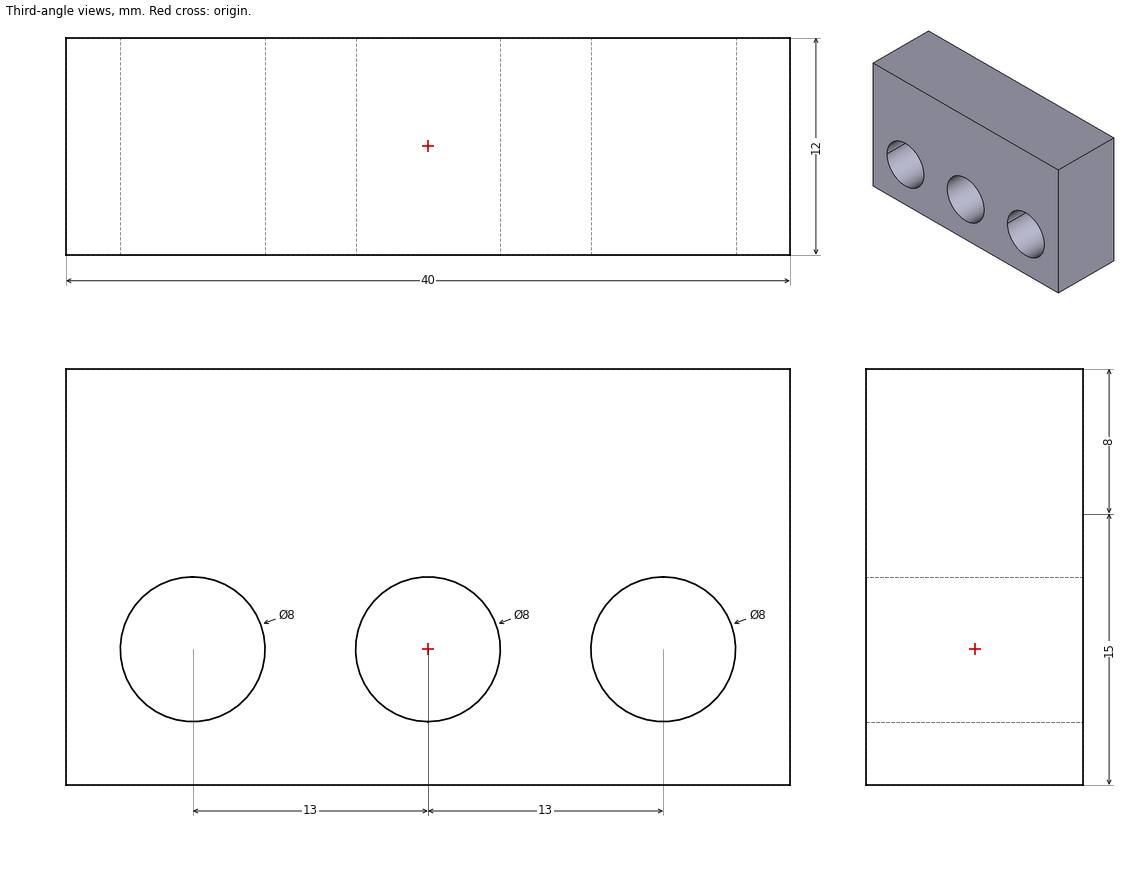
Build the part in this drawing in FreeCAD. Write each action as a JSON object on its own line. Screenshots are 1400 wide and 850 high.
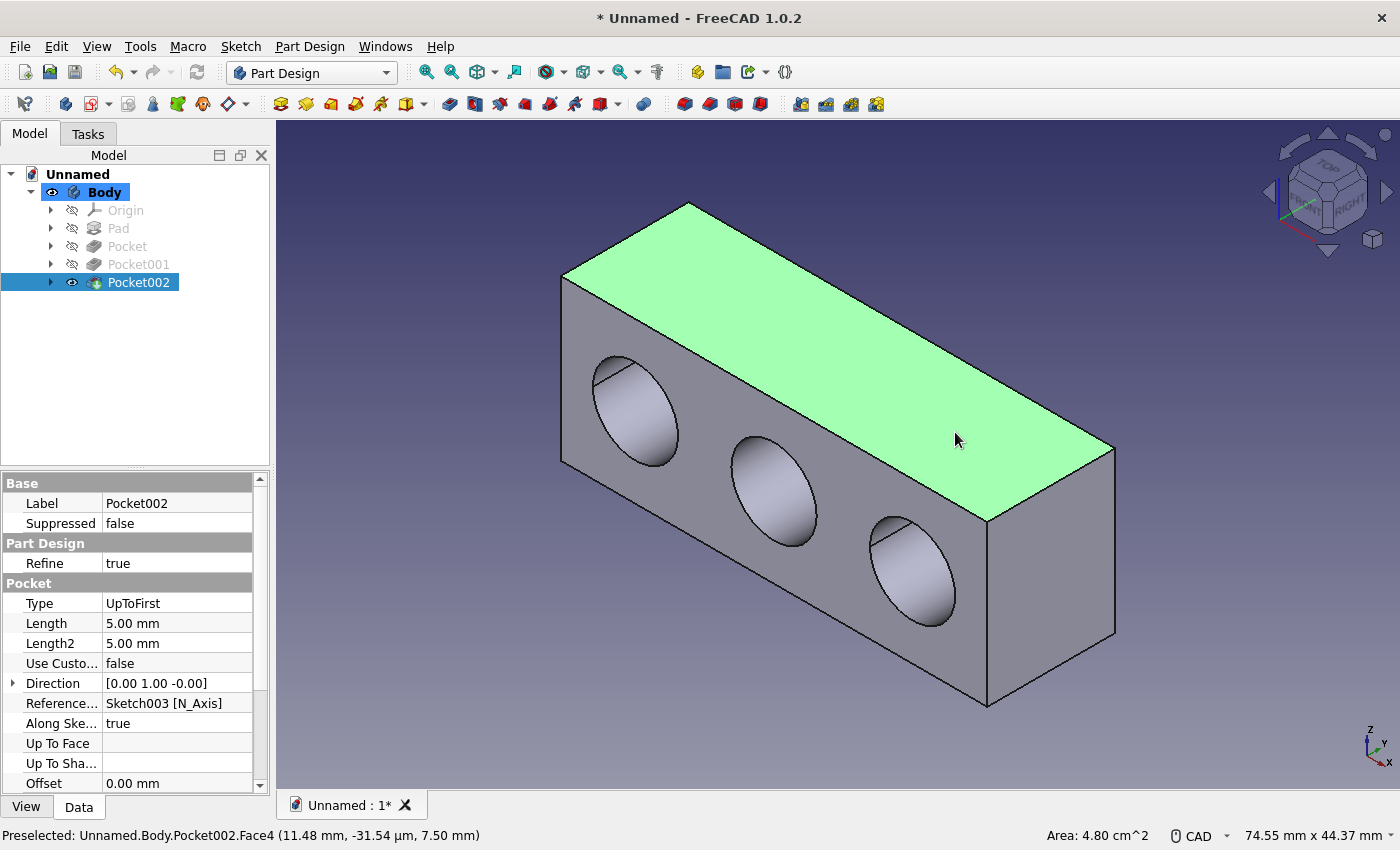
{"action": "left_click", "coordinate": [90, 104]}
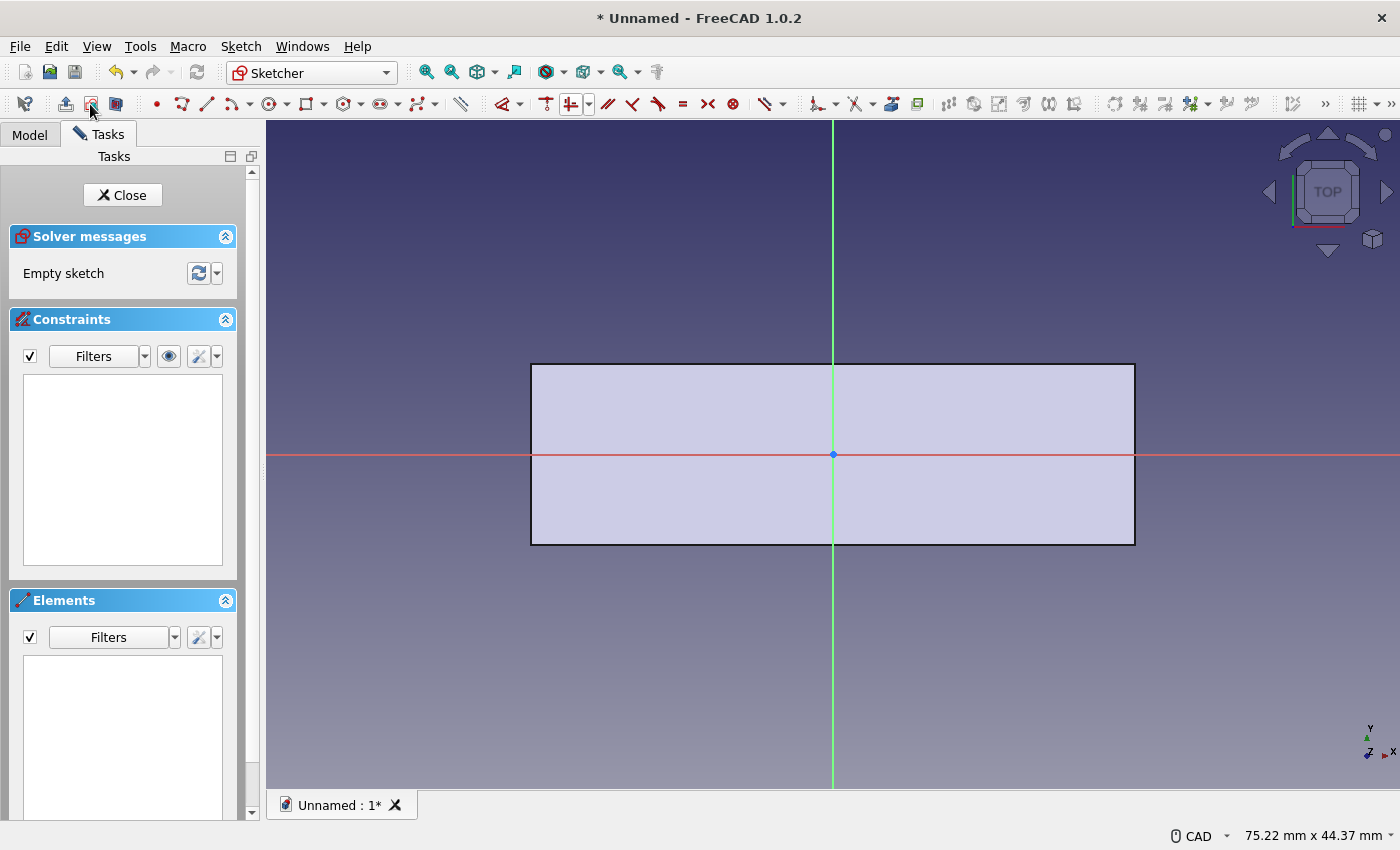
{"action": "key", "text": "g v"}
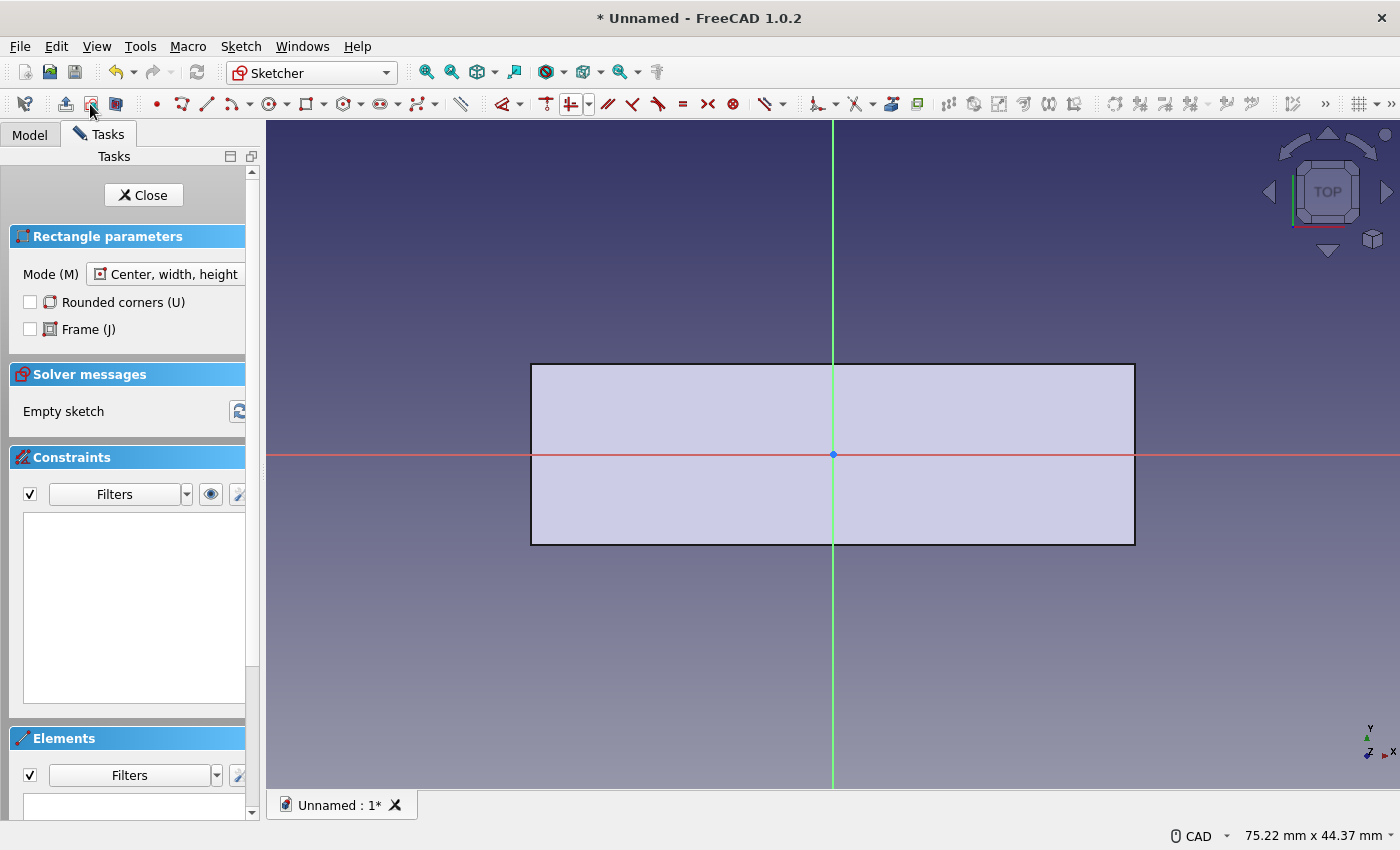
{"action": "left_click", "coordinate": [833, 454]}
{"action": "left_click", "coordinate": [1135, 364]}
{"action": "key", "text": "Escape"}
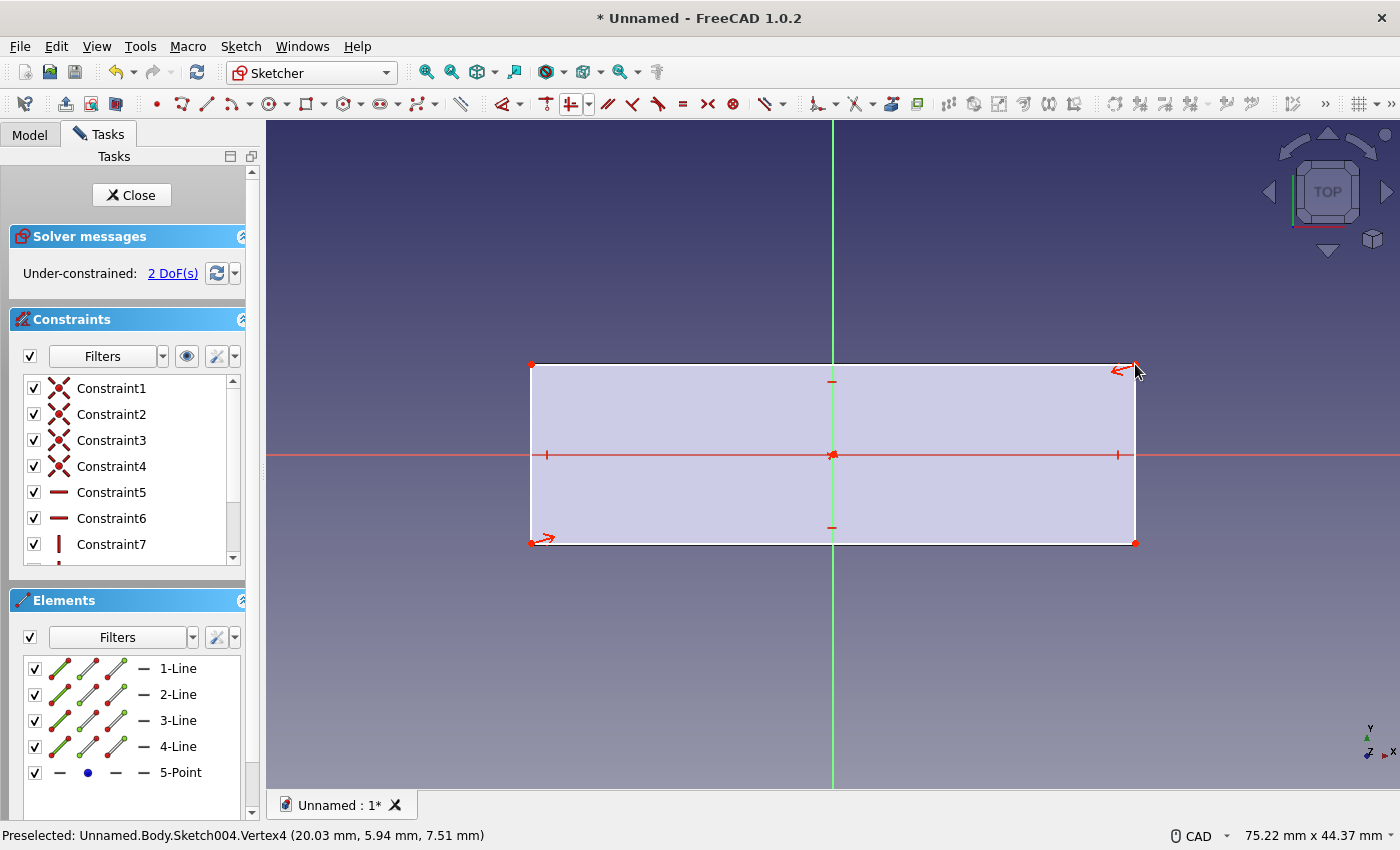
{"action": "left_click", "coordinate": [502, 104]}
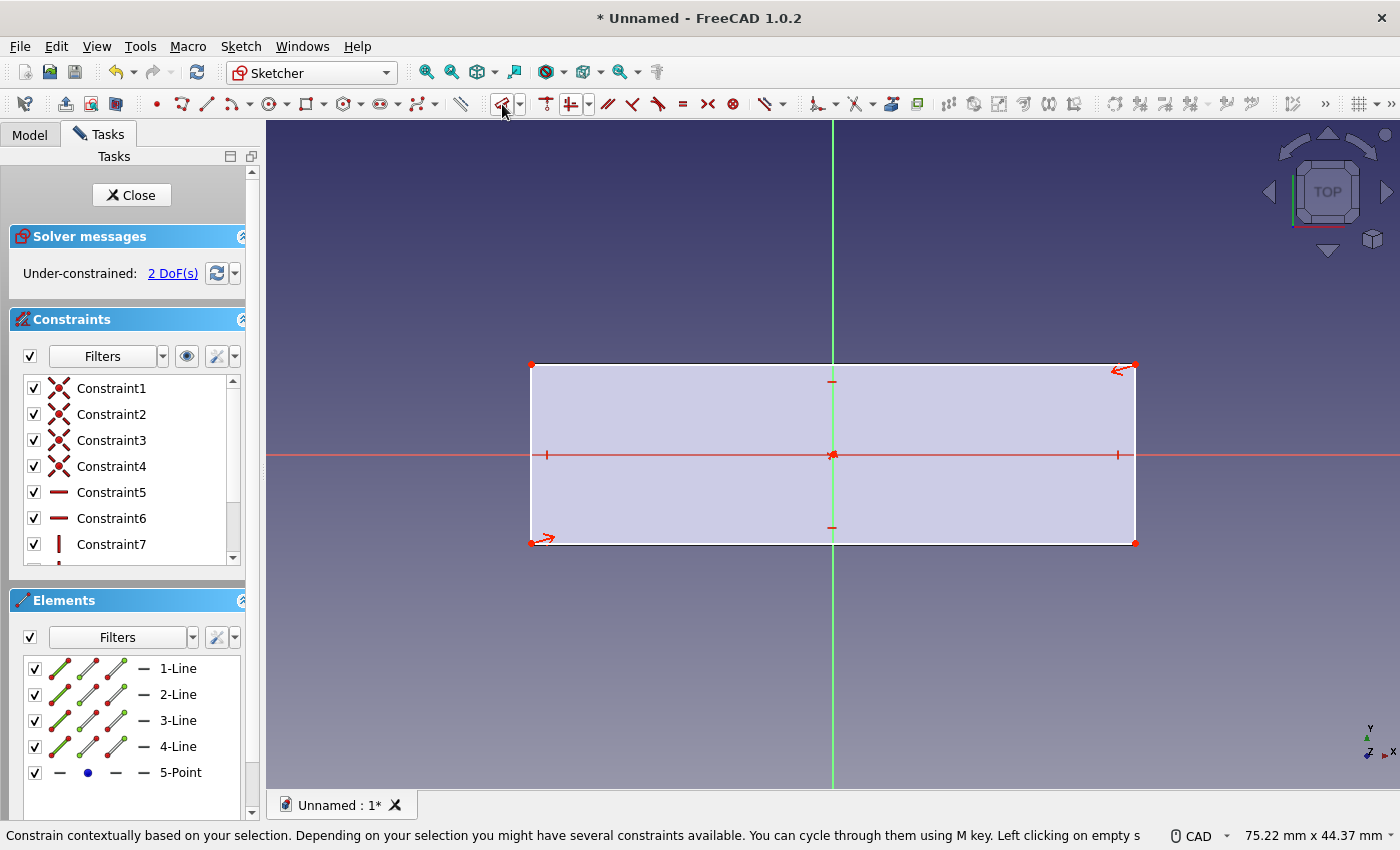
{"action": "left_click", "coordinate": [712, 544]}
{"action": "left_click", "coordinate": [694, 578]}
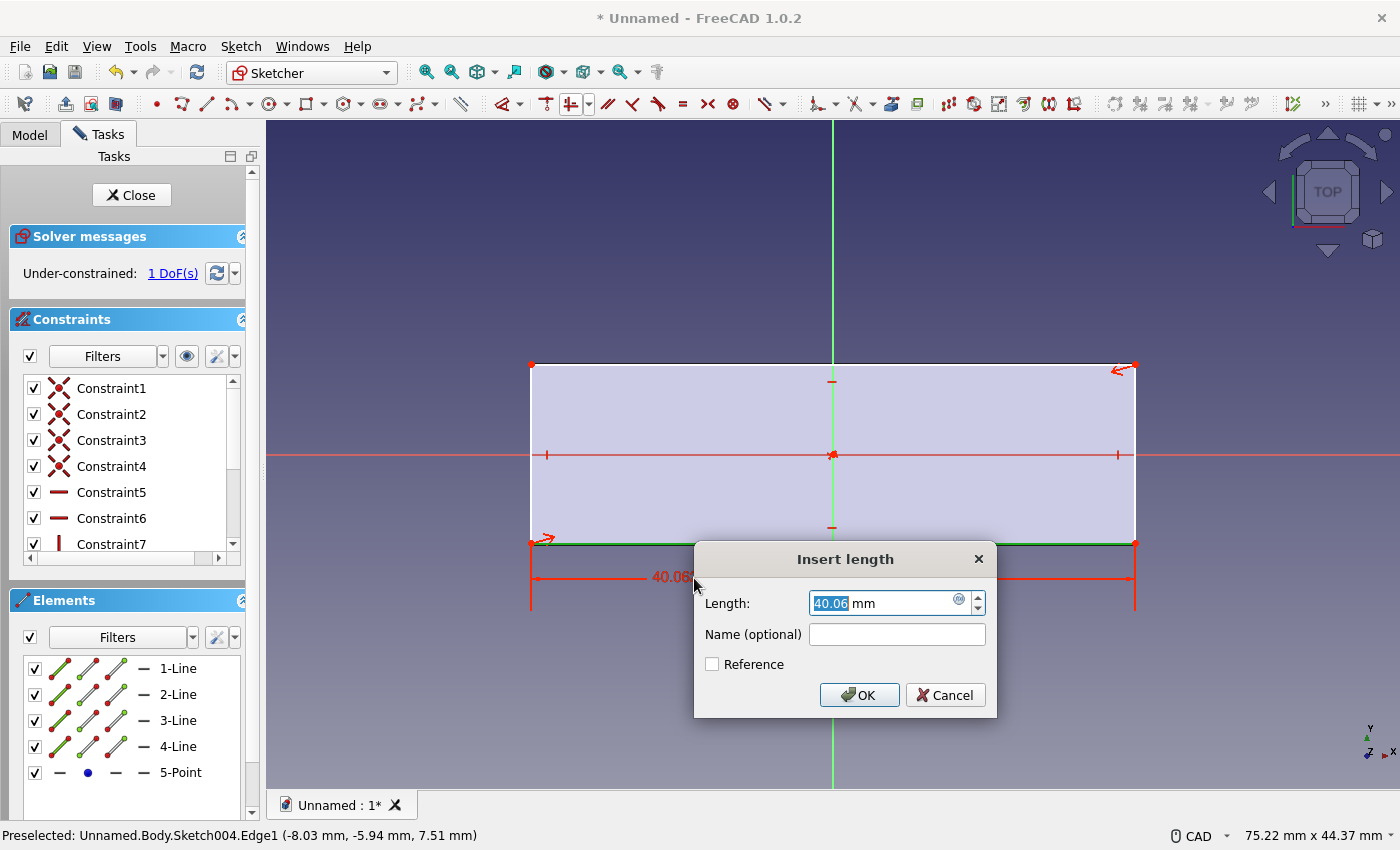
{"action": "type", "text": "40"}
{"action": "key", "text": "Return"}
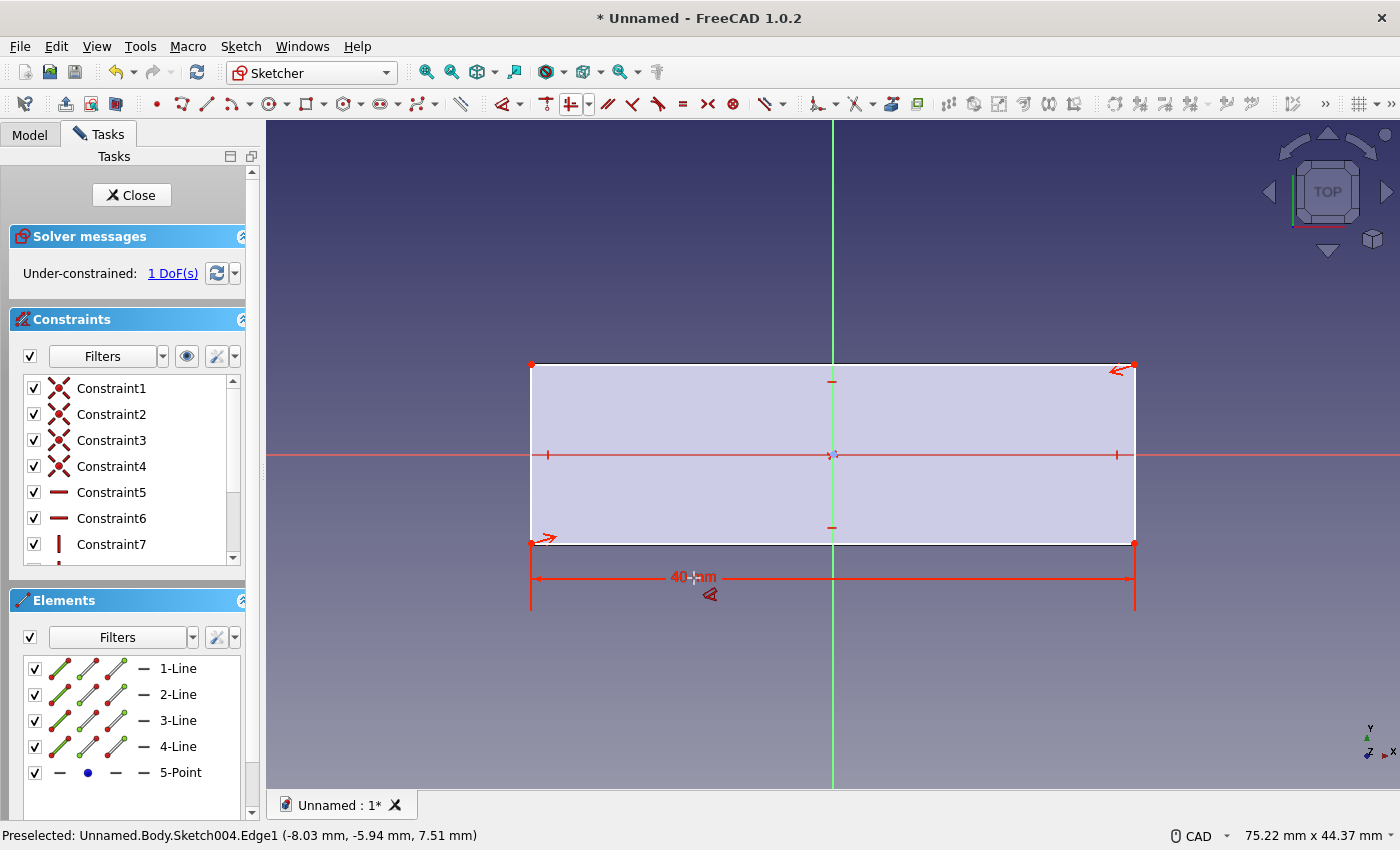
{"action": "left_click", "coordinate": [1135, 490]}
{"action": "left_click", "coordinate": [1169, 413]}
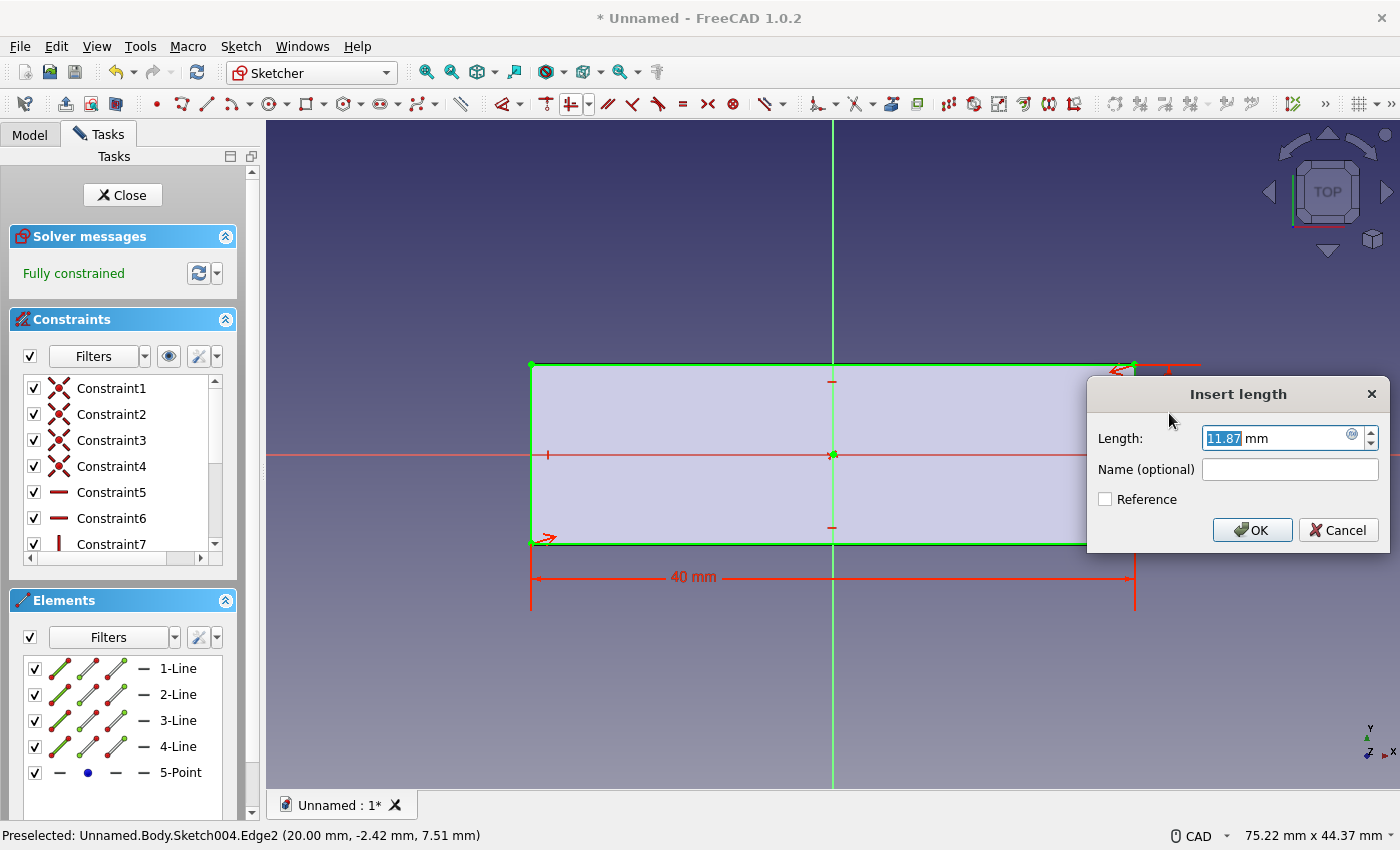
{"action": "type", "text": "12"}
{"action": "key", "text": "Return"}
{"action": "key", "text": "Escape"}